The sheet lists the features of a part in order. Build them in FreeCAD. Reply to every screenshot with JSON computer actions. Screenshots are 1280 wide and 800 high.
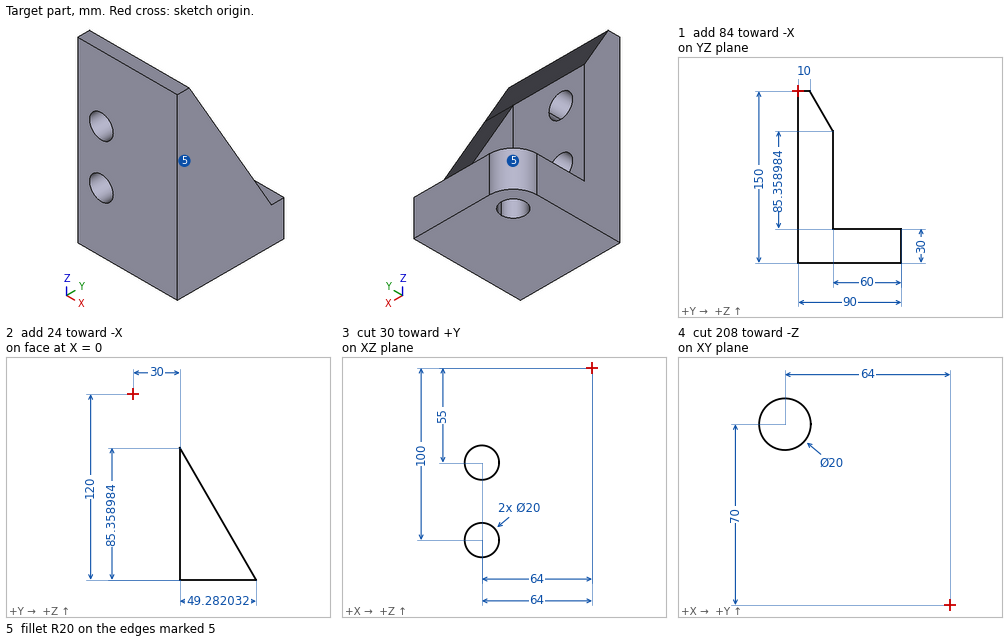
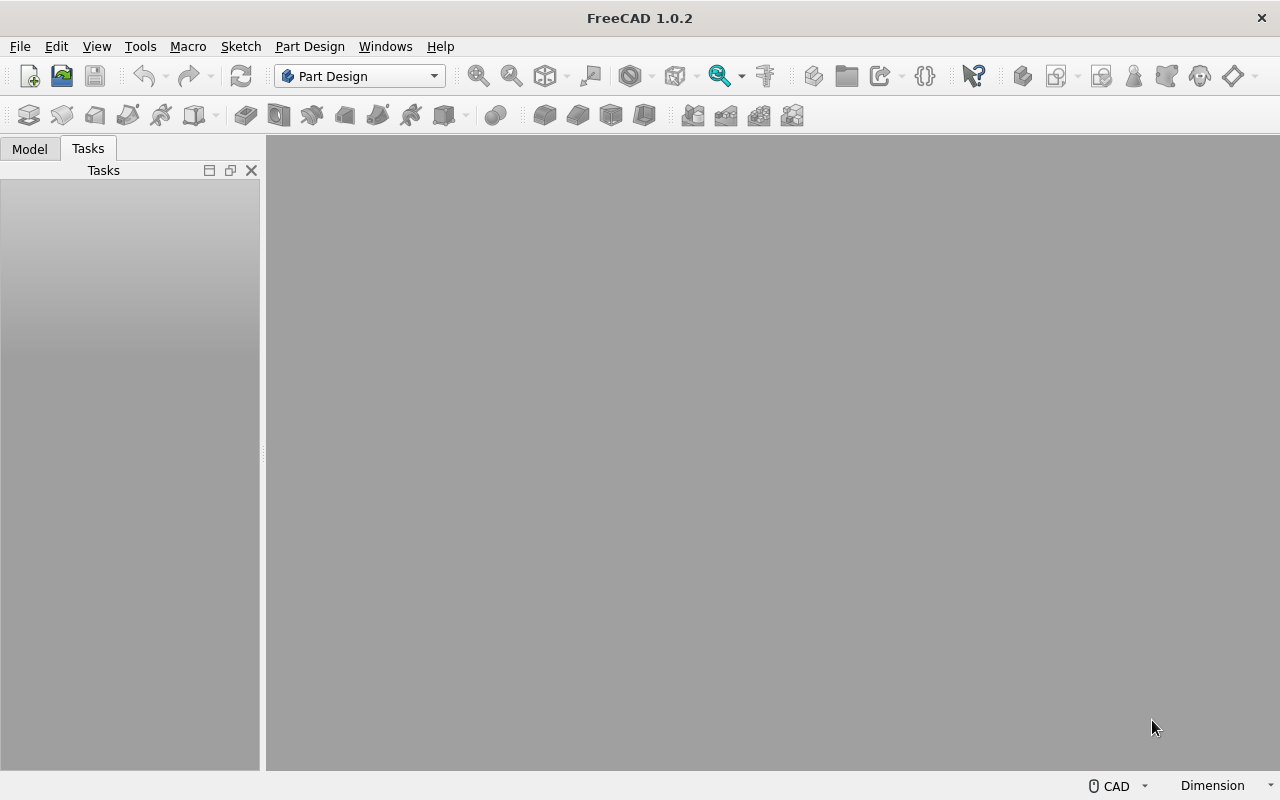
{"action": "left_click", "coordinate": [29, 76]}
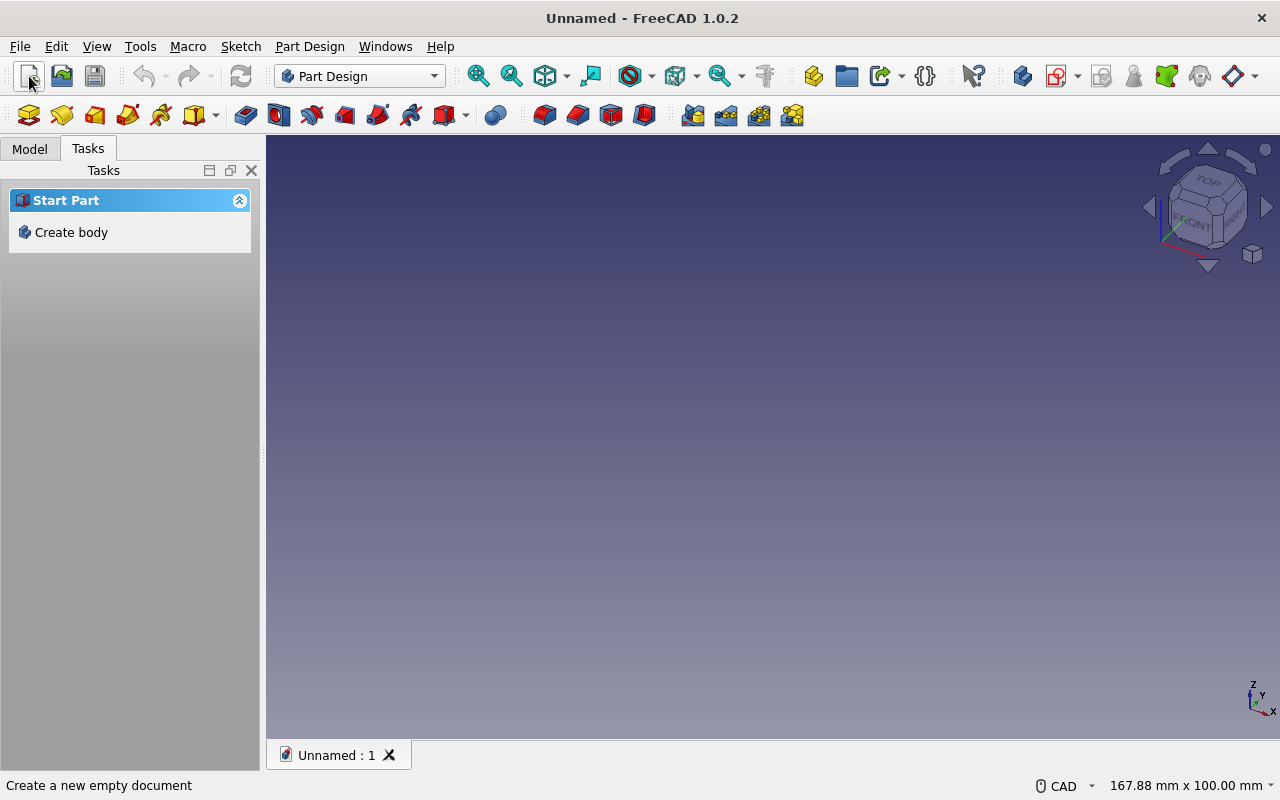
{"action": "left_click", "coordinate": [1056, 76]}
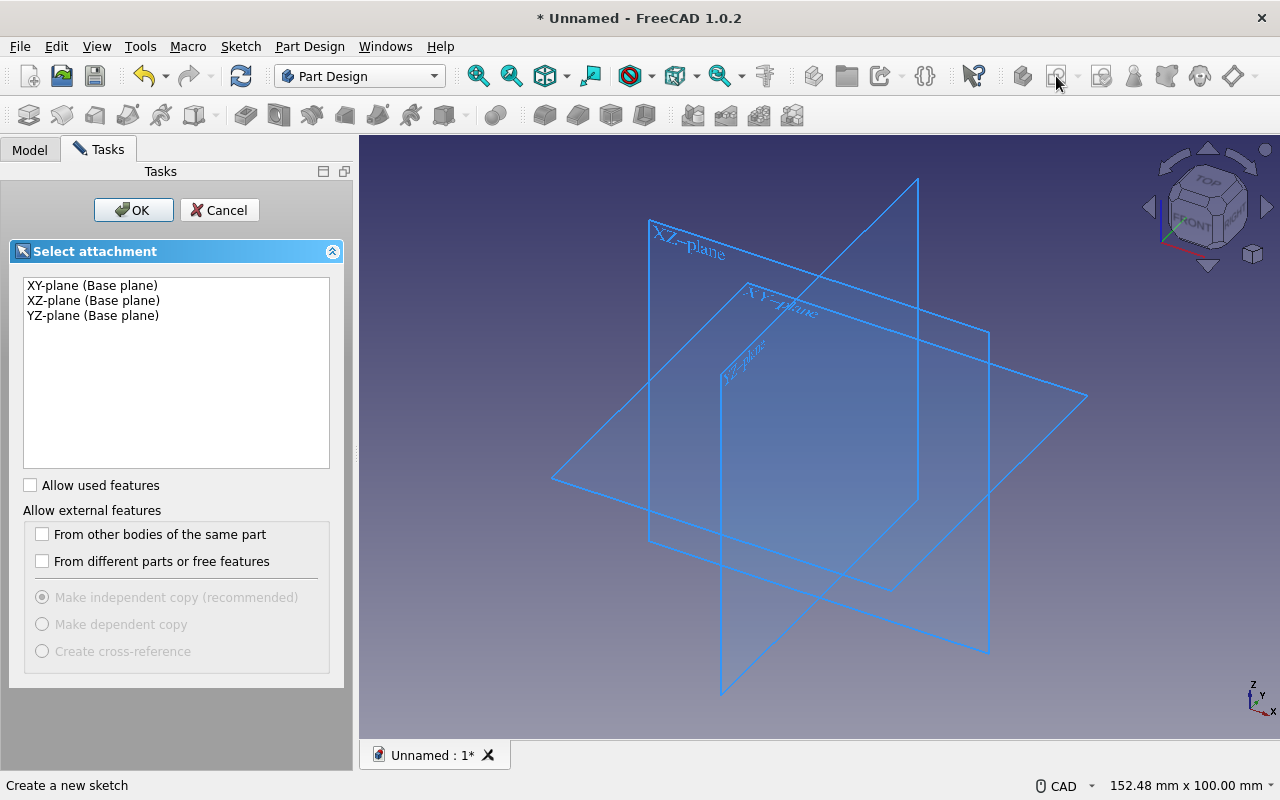
{"action": "left_click", "coordinate": [84, 316]}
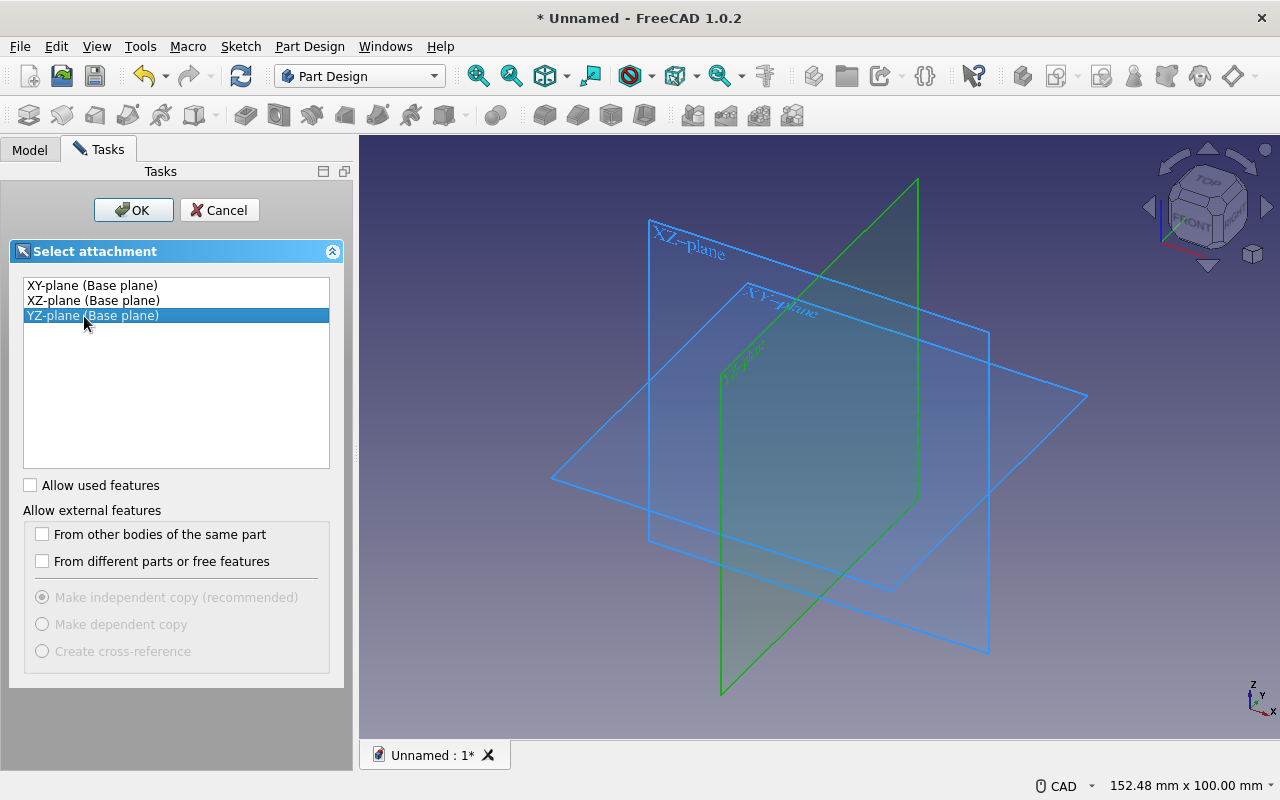
{"action": "left_click", "coordinate": [134, 210]}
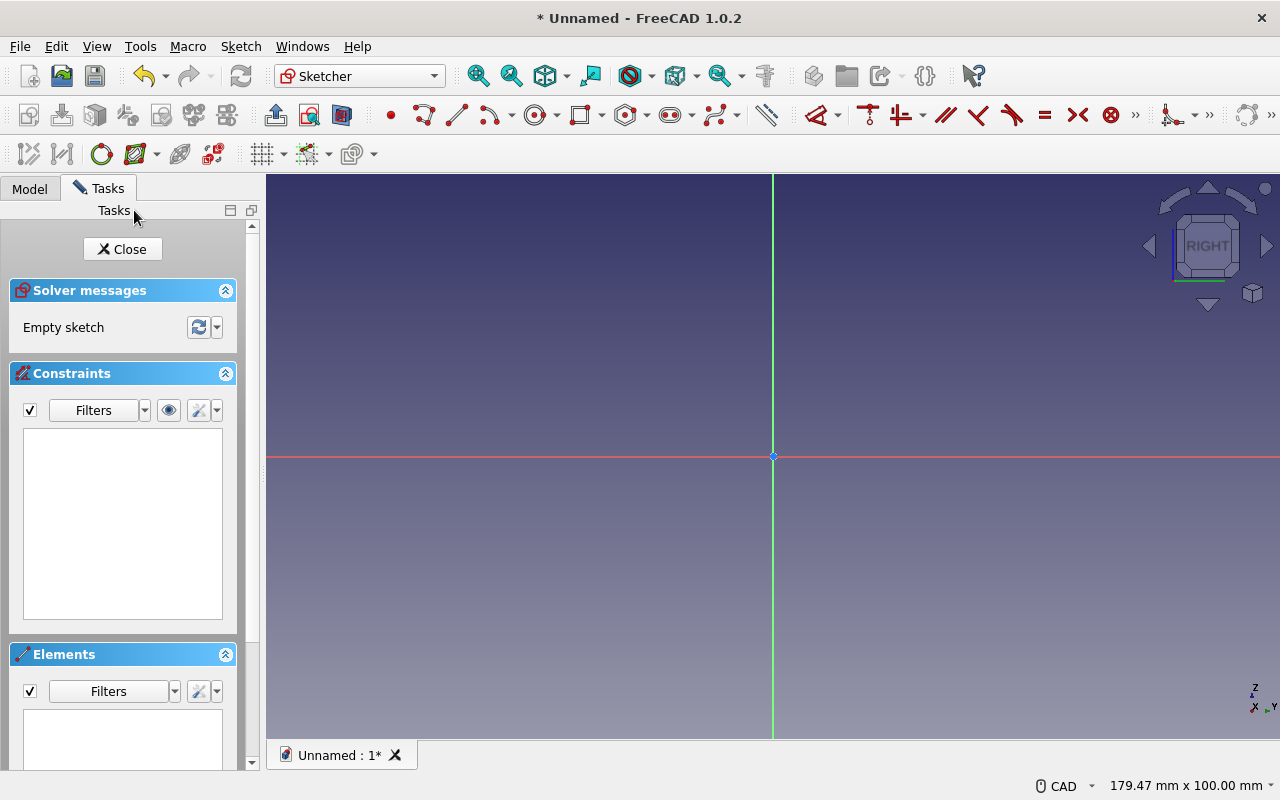
{"action": "scroll", "coordinate": [517, 210], "scroll_direction": "down", "scroll_amount": 5}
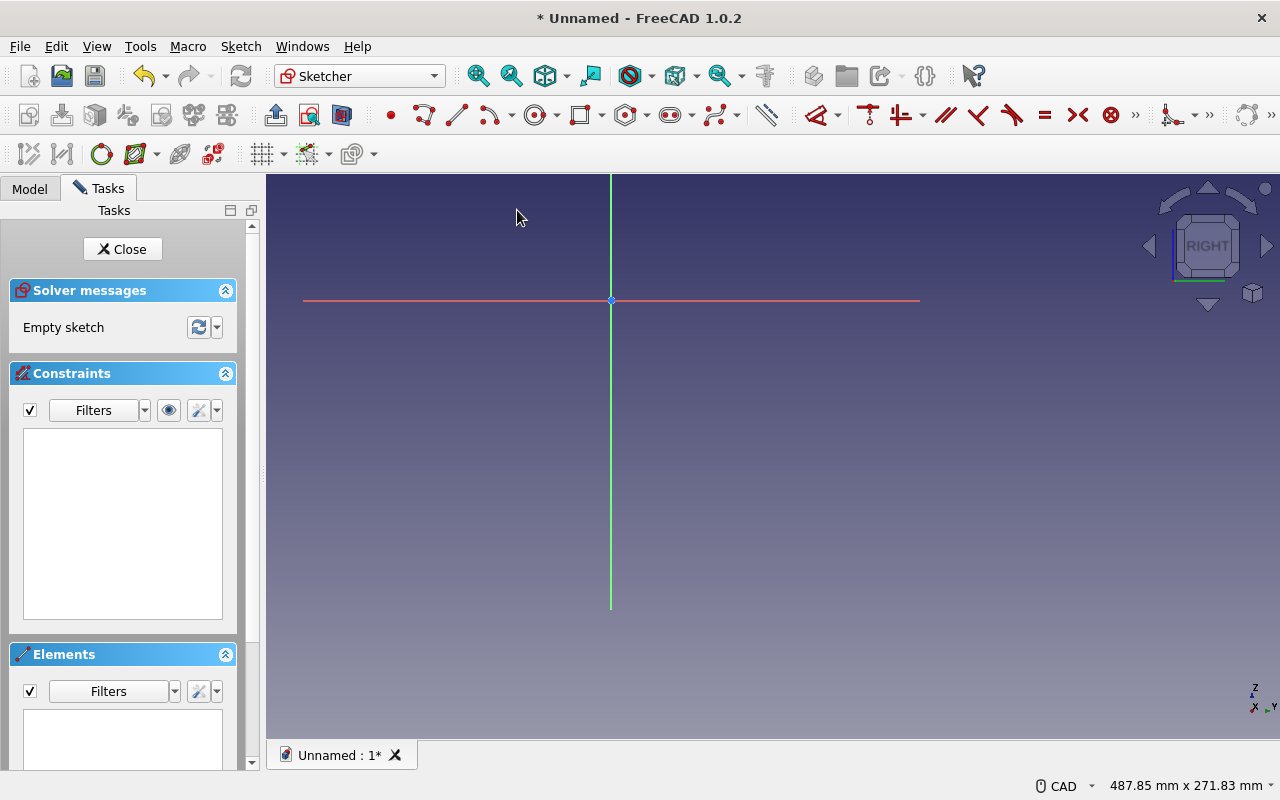
{"action": "left_click", "coordinate": [424, 116]}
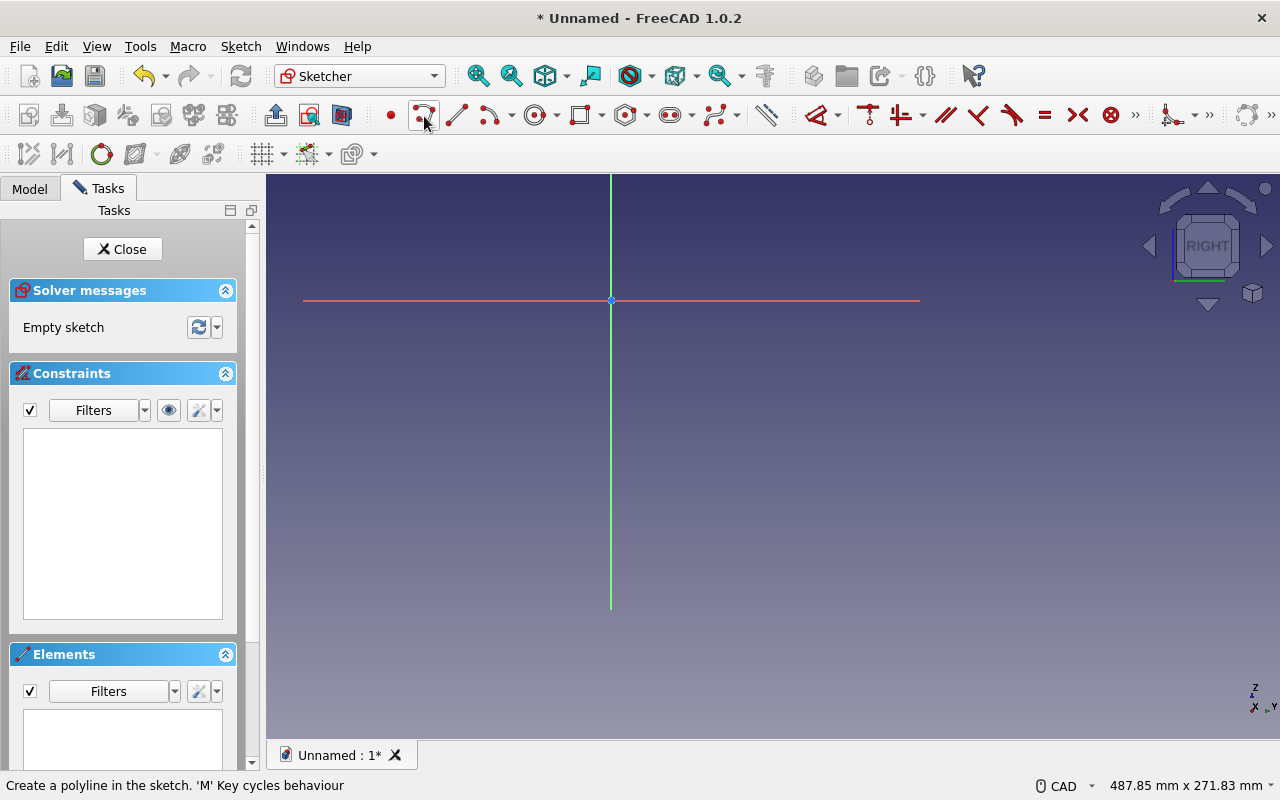
{"action": "left_click", "coordinate": [611, 301]}
{"action": "left_click", "coordinate": [620, 613]}
{"action": "left_click", "coordinate": [798, 613]}
{"action": "left_click", "coordinate": [798, 550]}
{"action": "left_click", "coordinate": [674, 550]}
{"action": "left_click", "coordinate": [674, 373]}
{"action": "left_click", "coordinate": [632, 310]}
{"action": "left_click", "coordinate": [611, 301]}
{"action": "key", "text": "Escape"}
{"action": "key", "text": "Escape"}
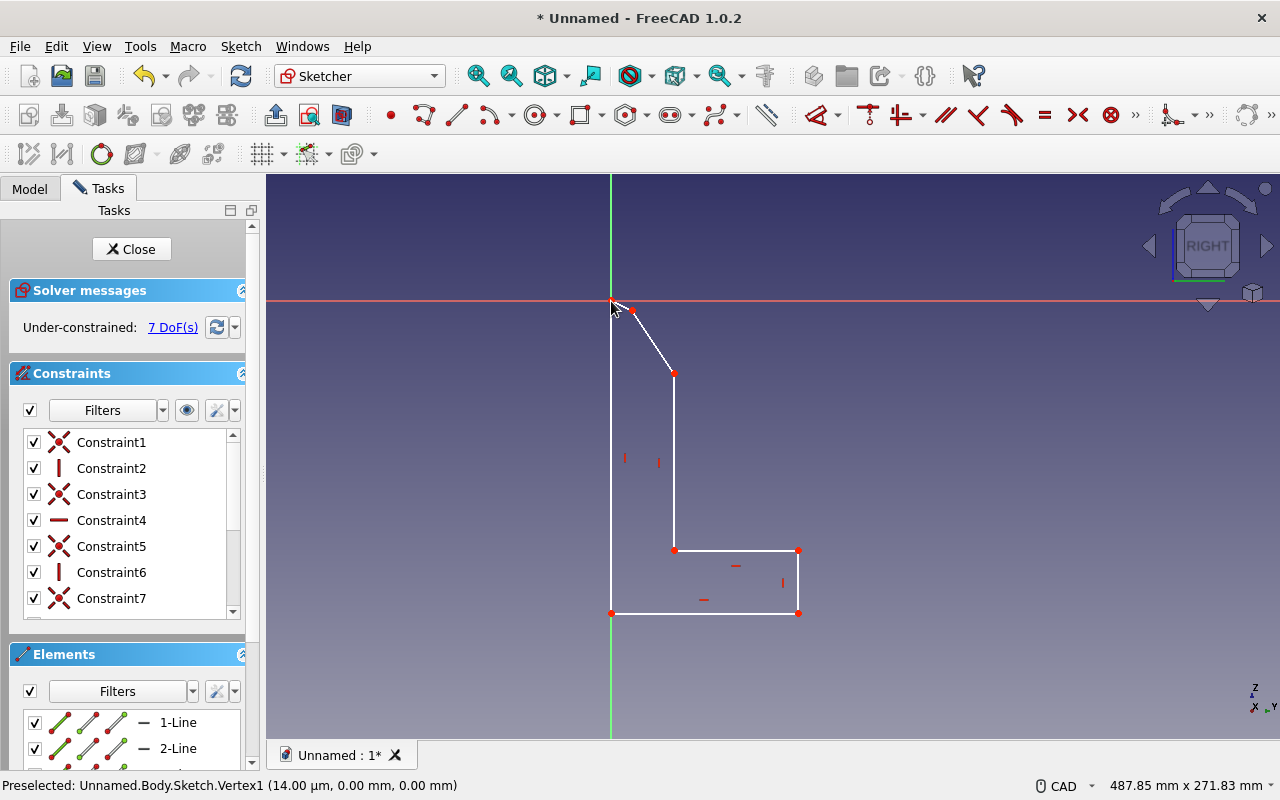
{"action": "scroll", "coordinate": [626, 308], "scroll_direction": "up", "scroll_amount": 4}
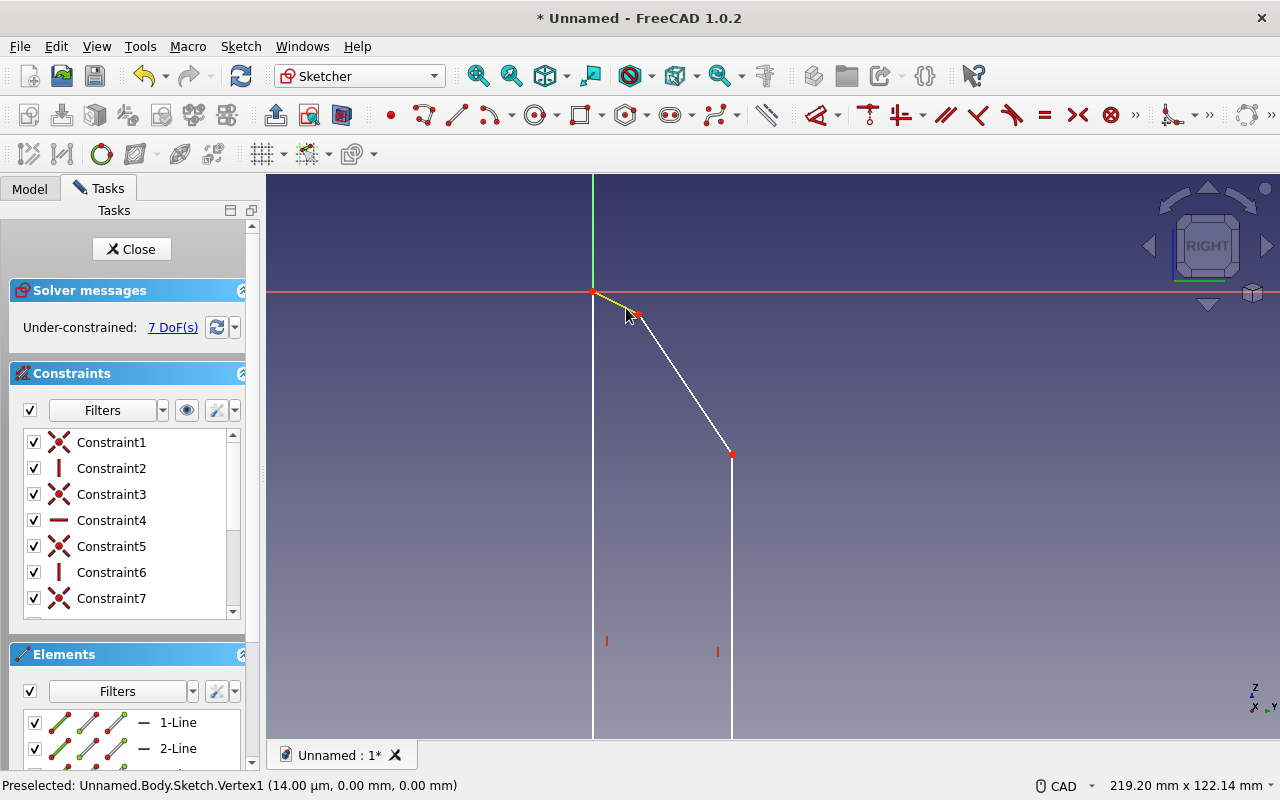
{"action": "left_click", "coordinate": [625, 308]}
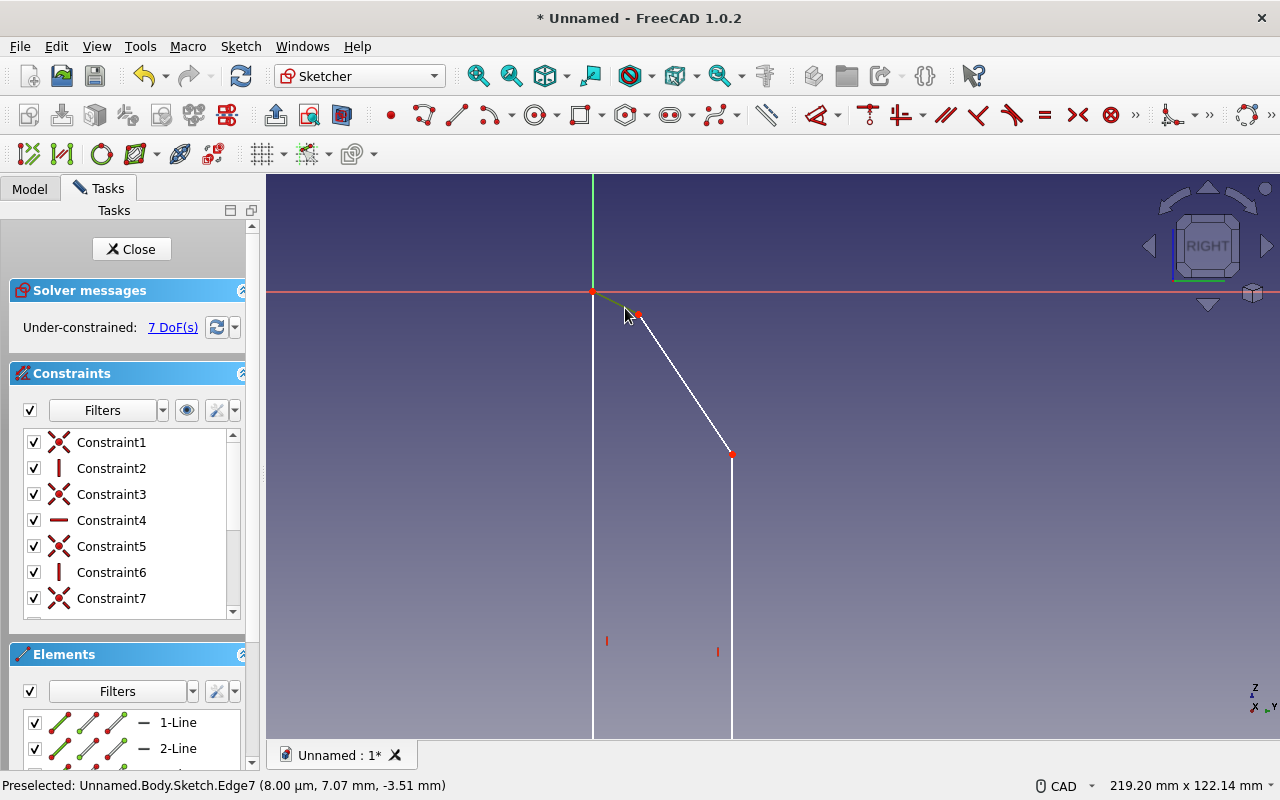
{"action": "key", "text": "h"}